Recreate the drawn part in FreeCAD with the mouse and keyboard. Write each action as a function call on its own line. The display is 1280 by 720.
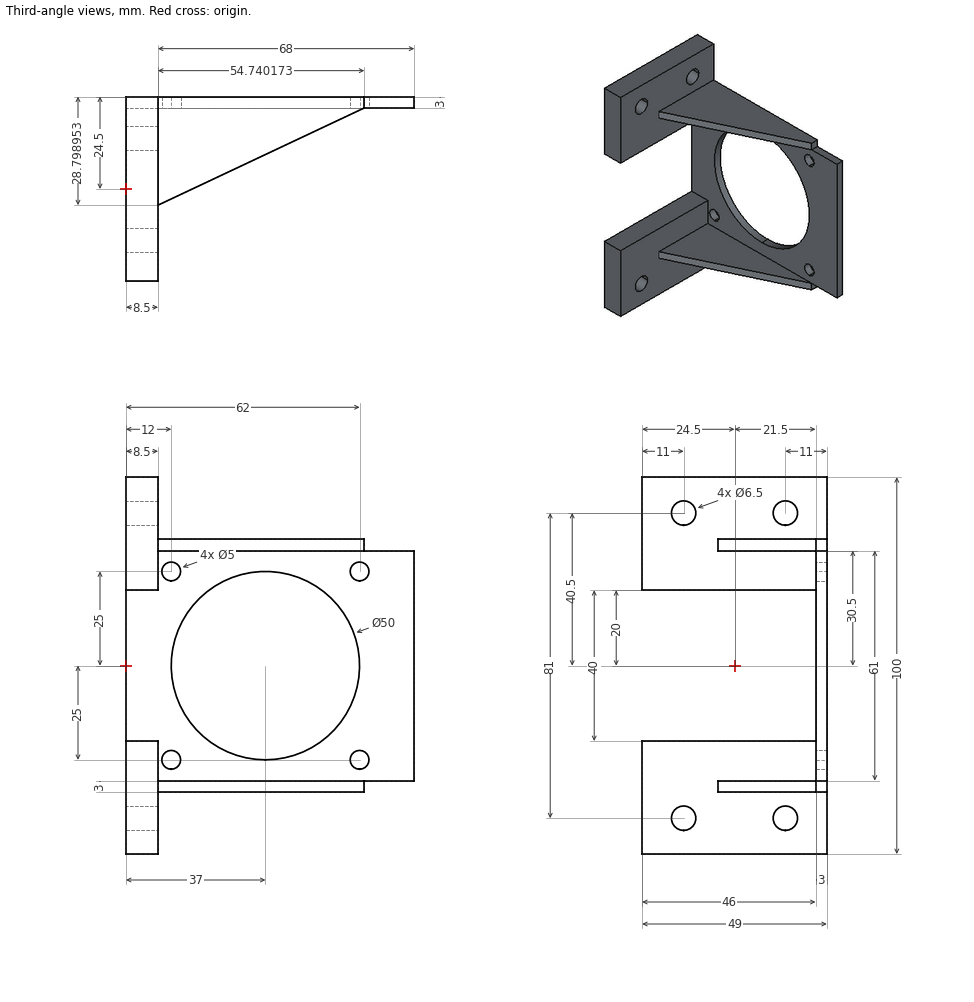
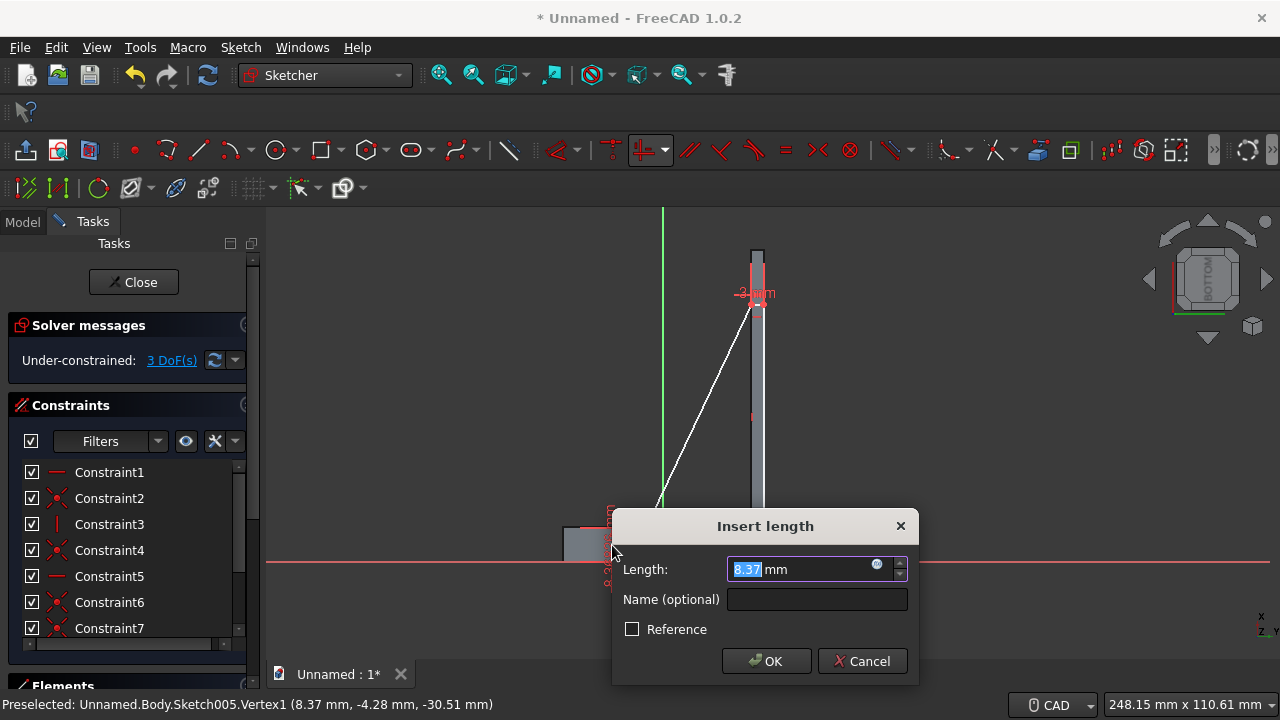
text(8.5)
key(Return)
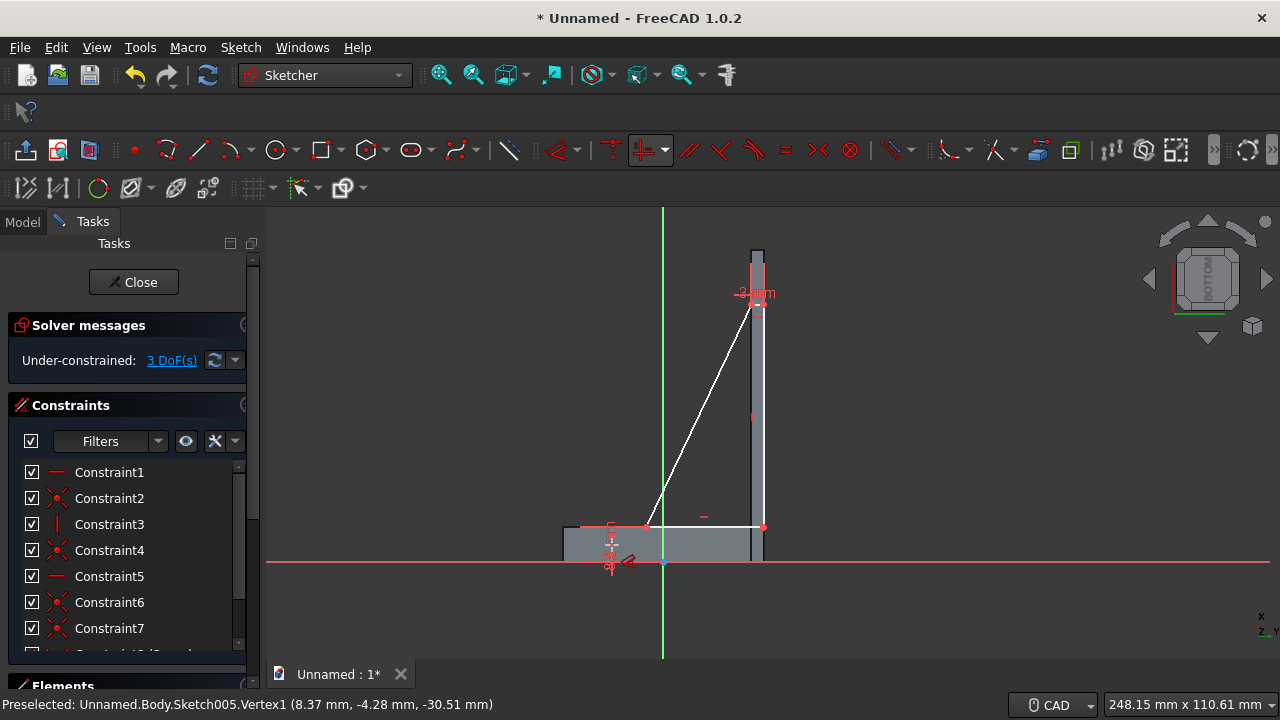
click(764, 527)
click(714, 596)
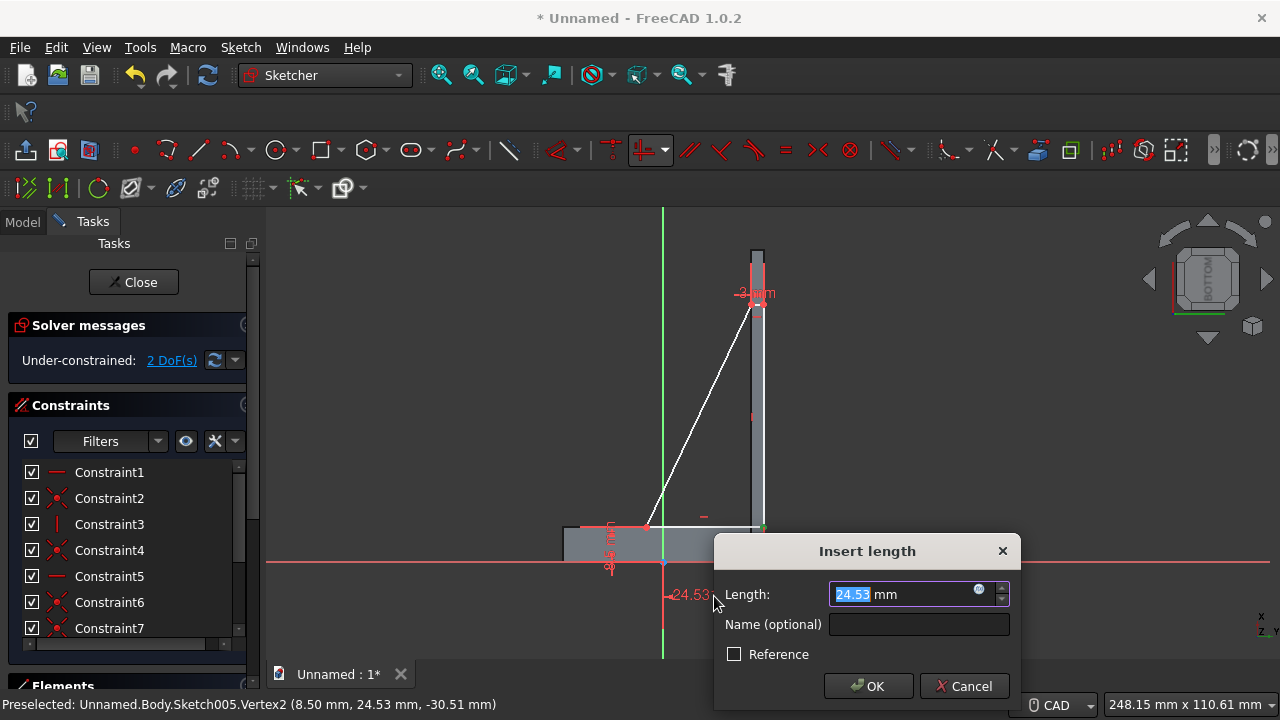
text(24.5)
key(Return)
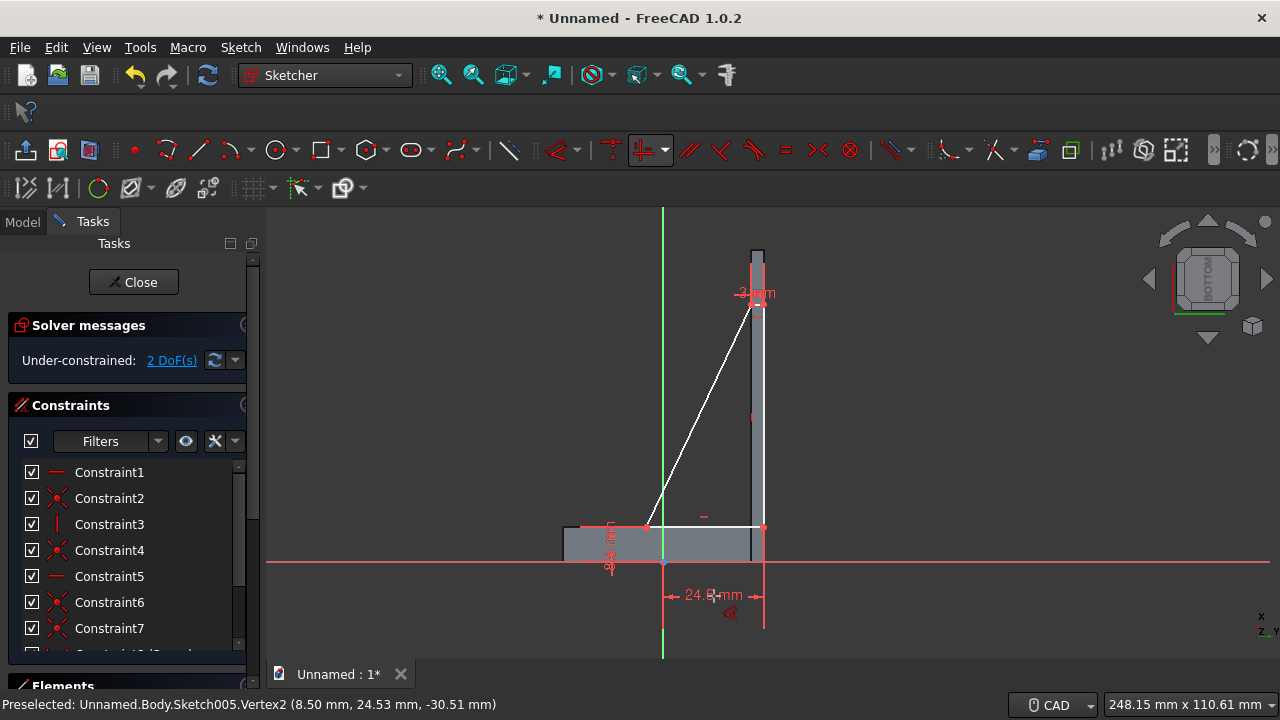
click(681, 527)
click(705, 493)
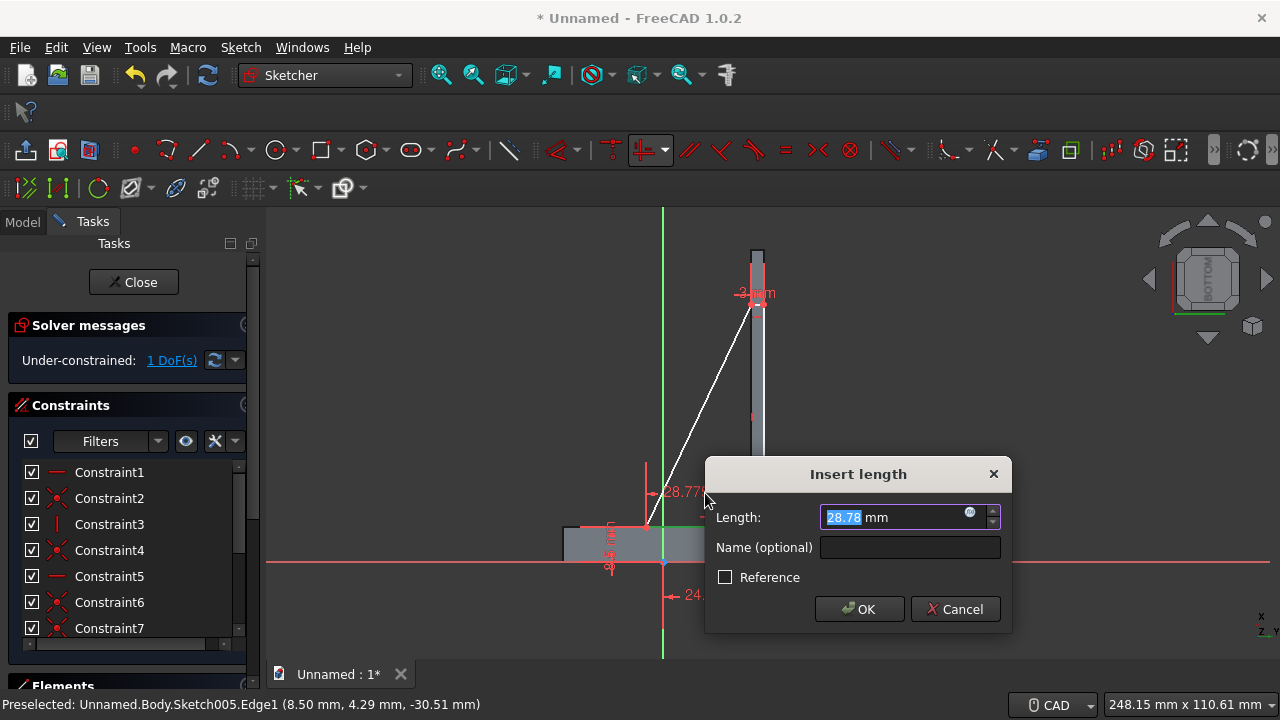
text(28.798953)
key(Return)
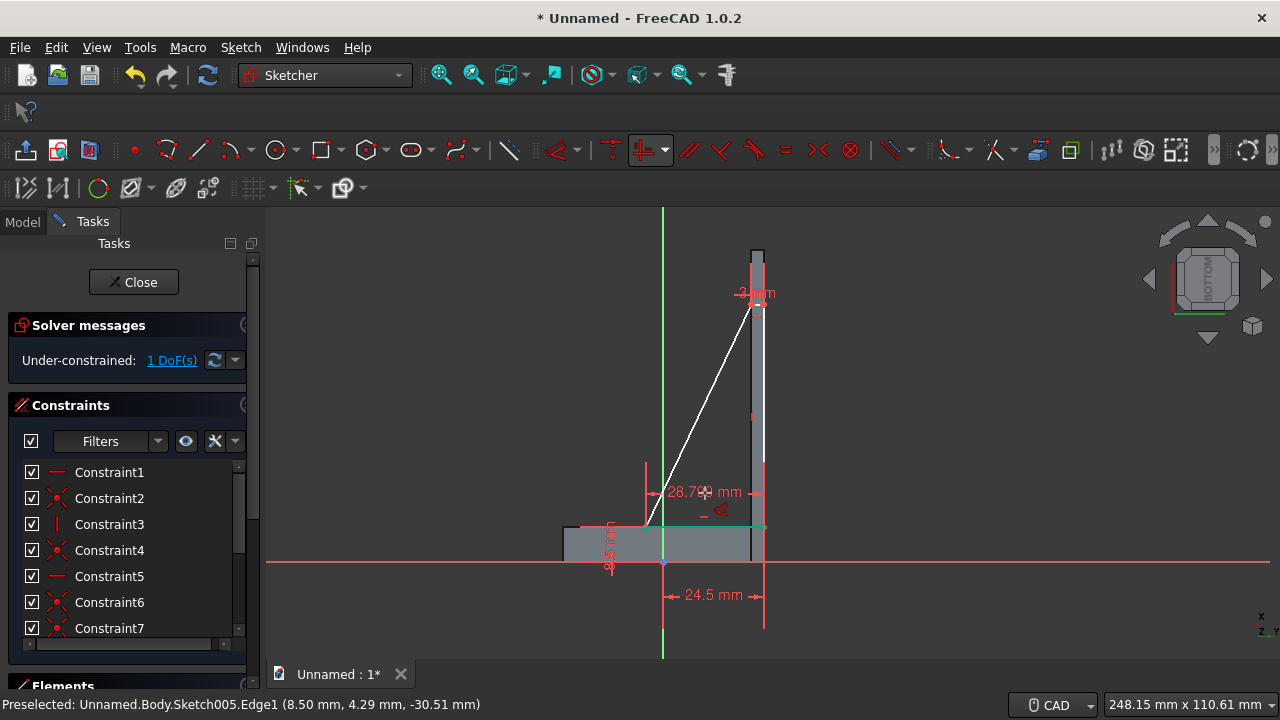
click(764, 461)
click(798, 416)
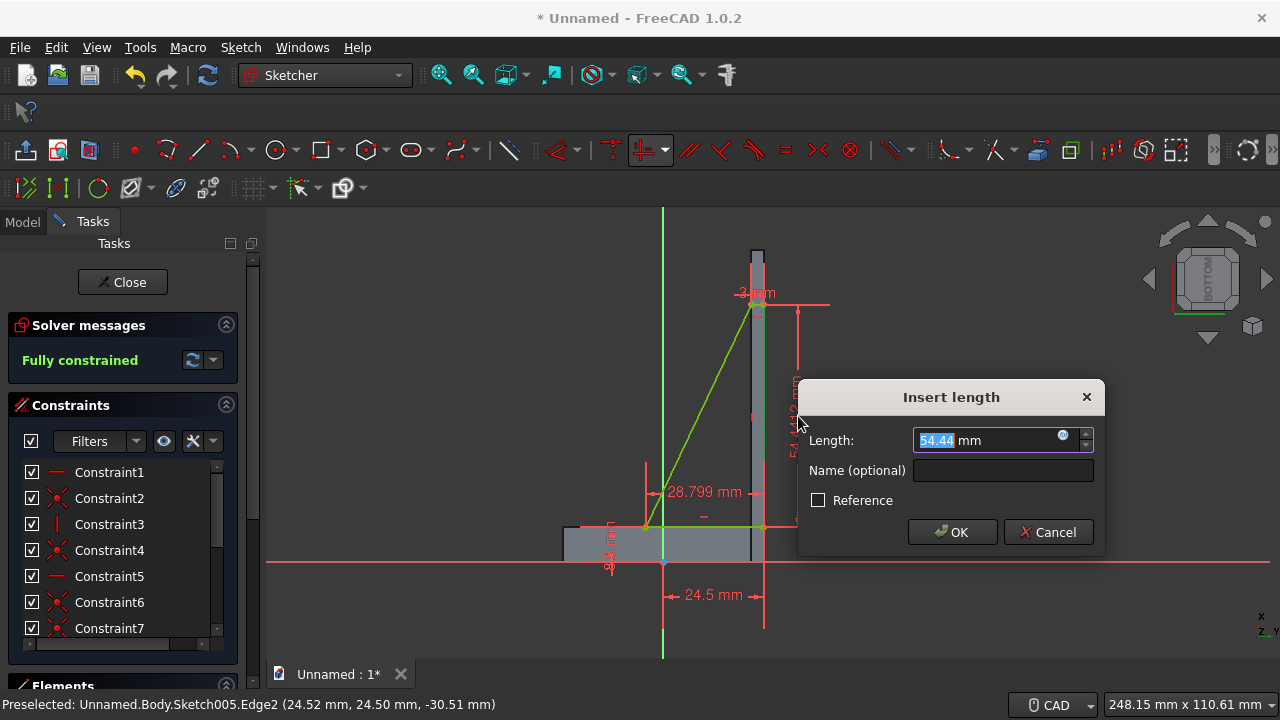
text(54.740173)
key(Return)
key(Escape)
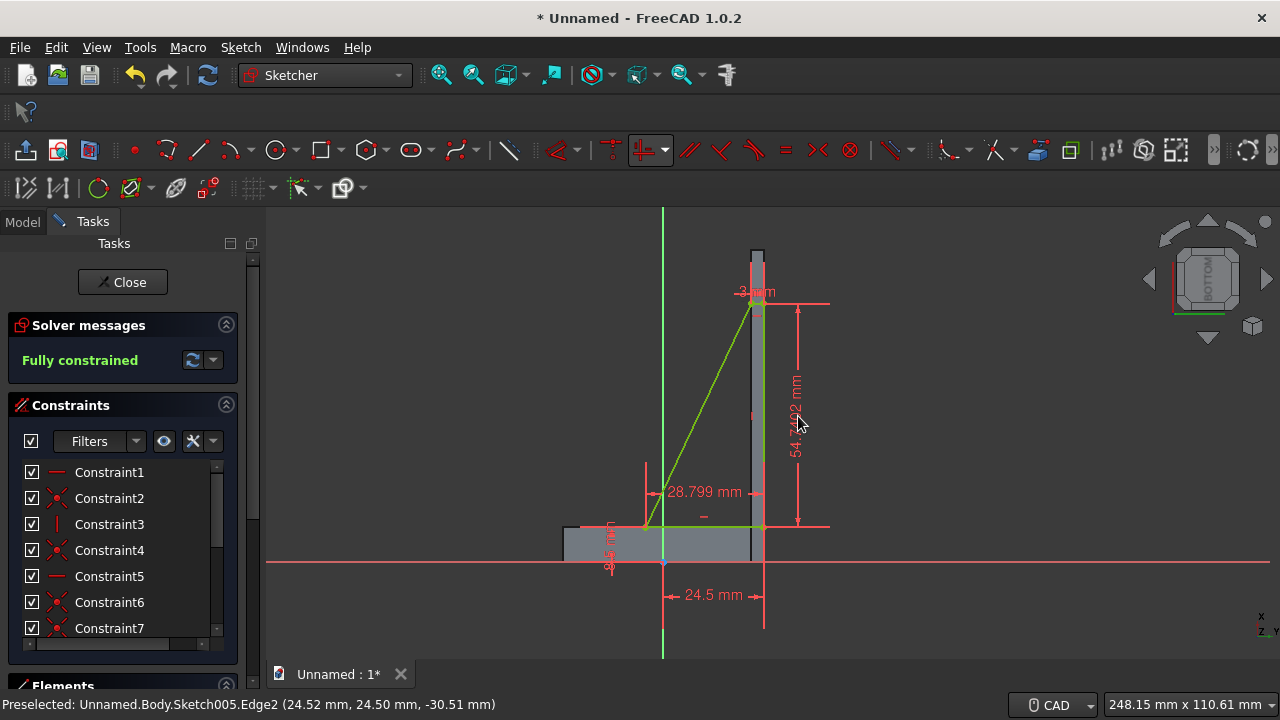
click(123, 282)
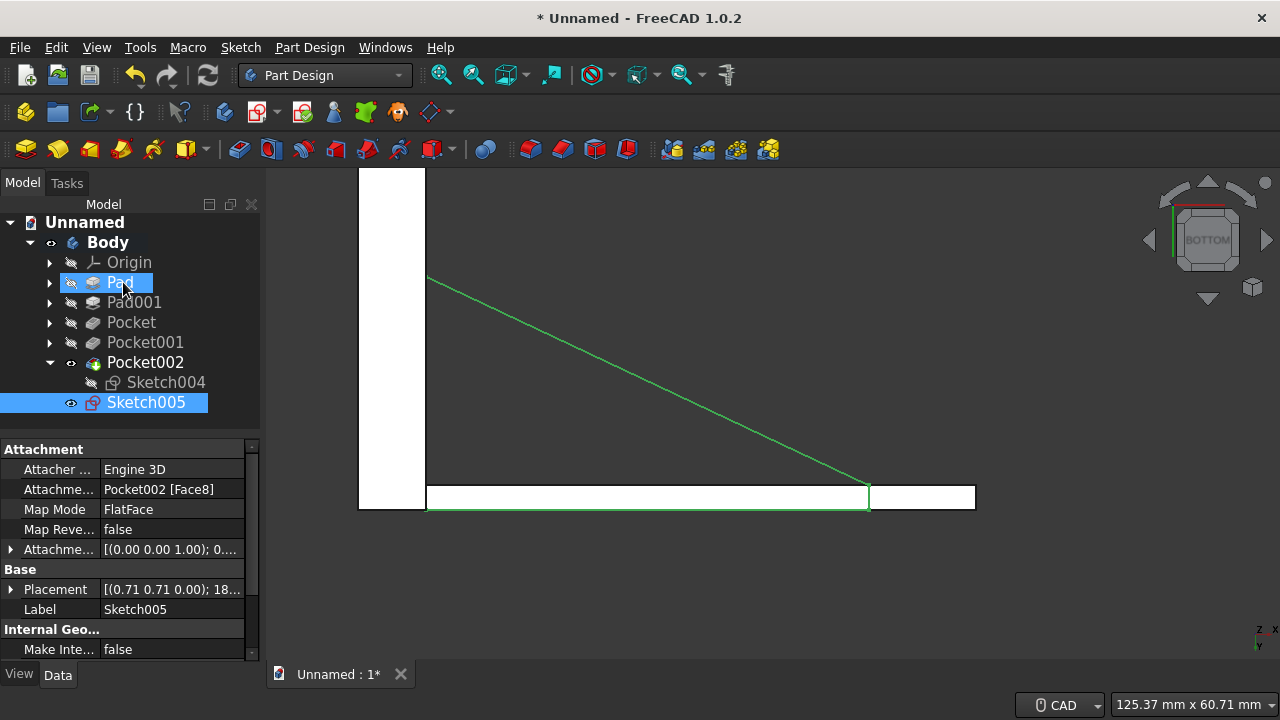
click(26, 150)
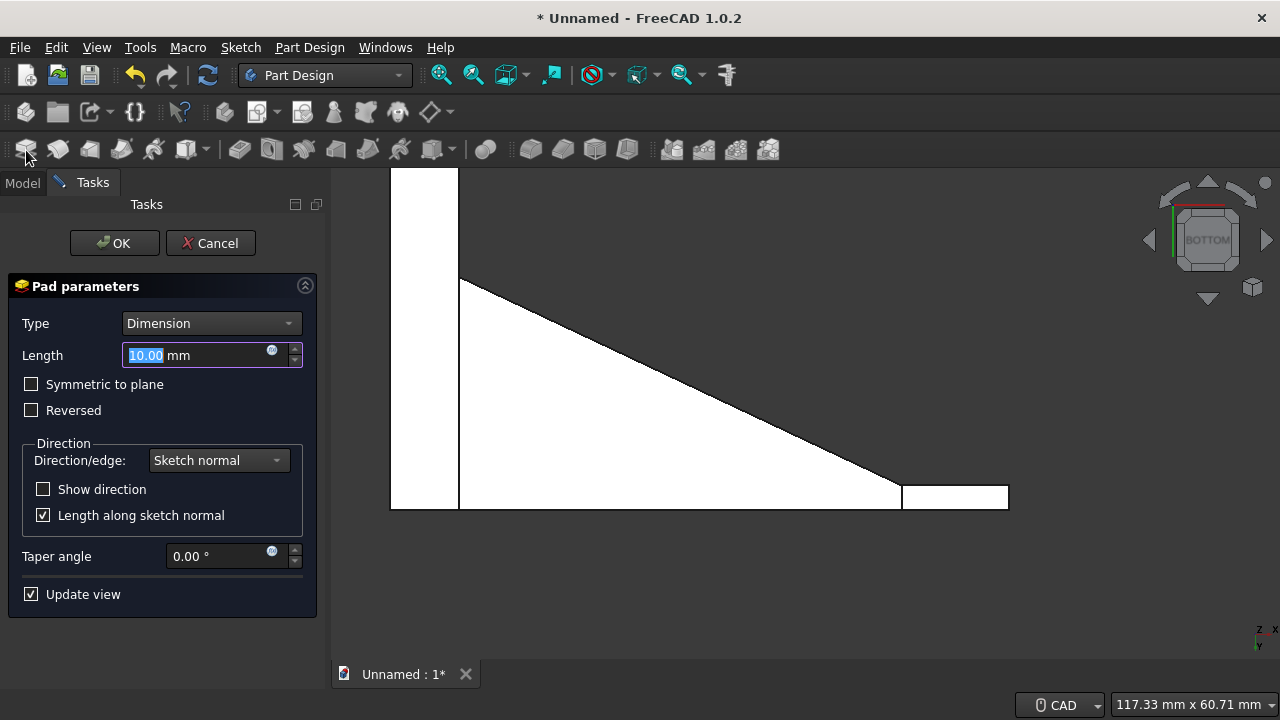
text(3)
key(Tab)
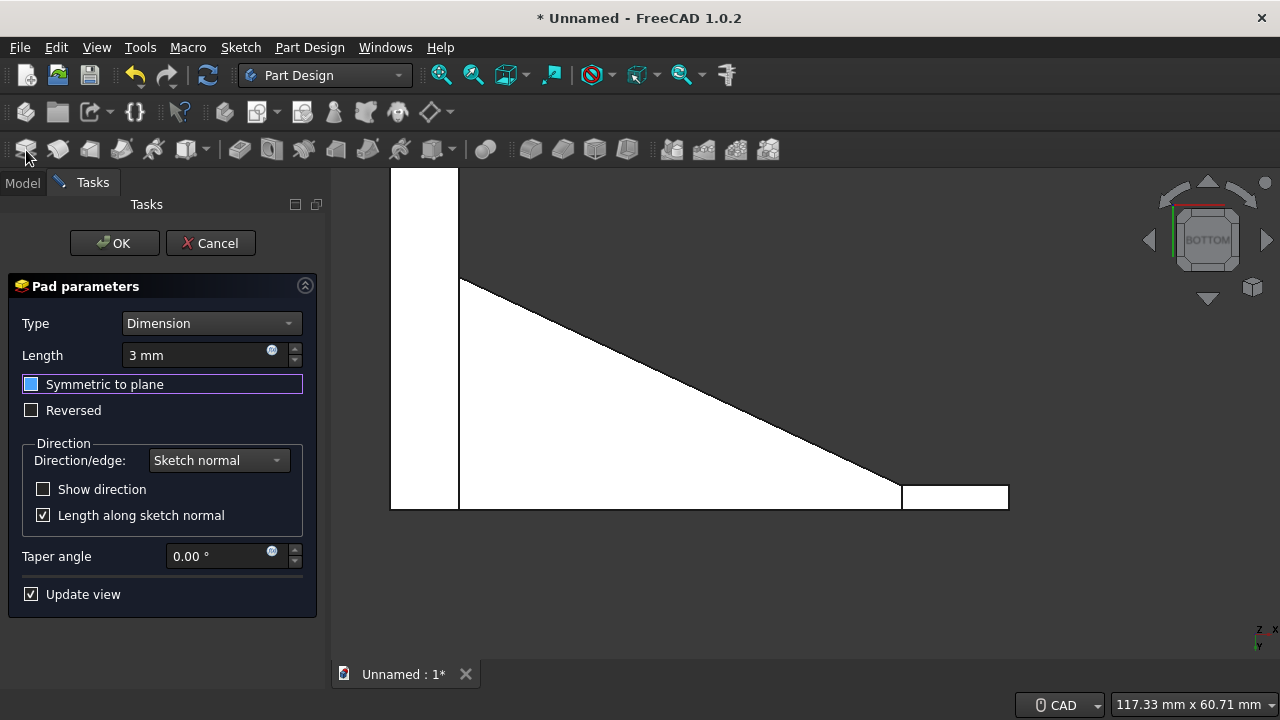
click(115, 243)